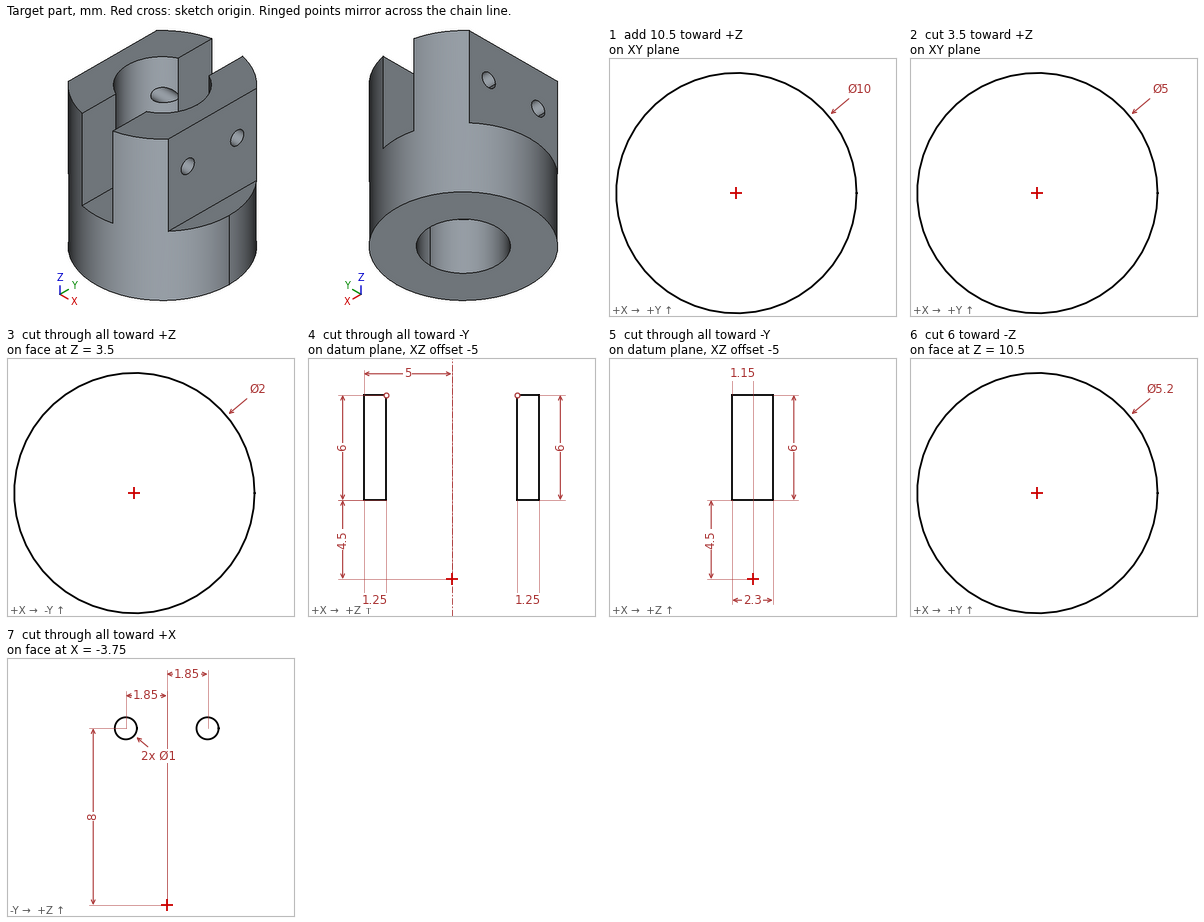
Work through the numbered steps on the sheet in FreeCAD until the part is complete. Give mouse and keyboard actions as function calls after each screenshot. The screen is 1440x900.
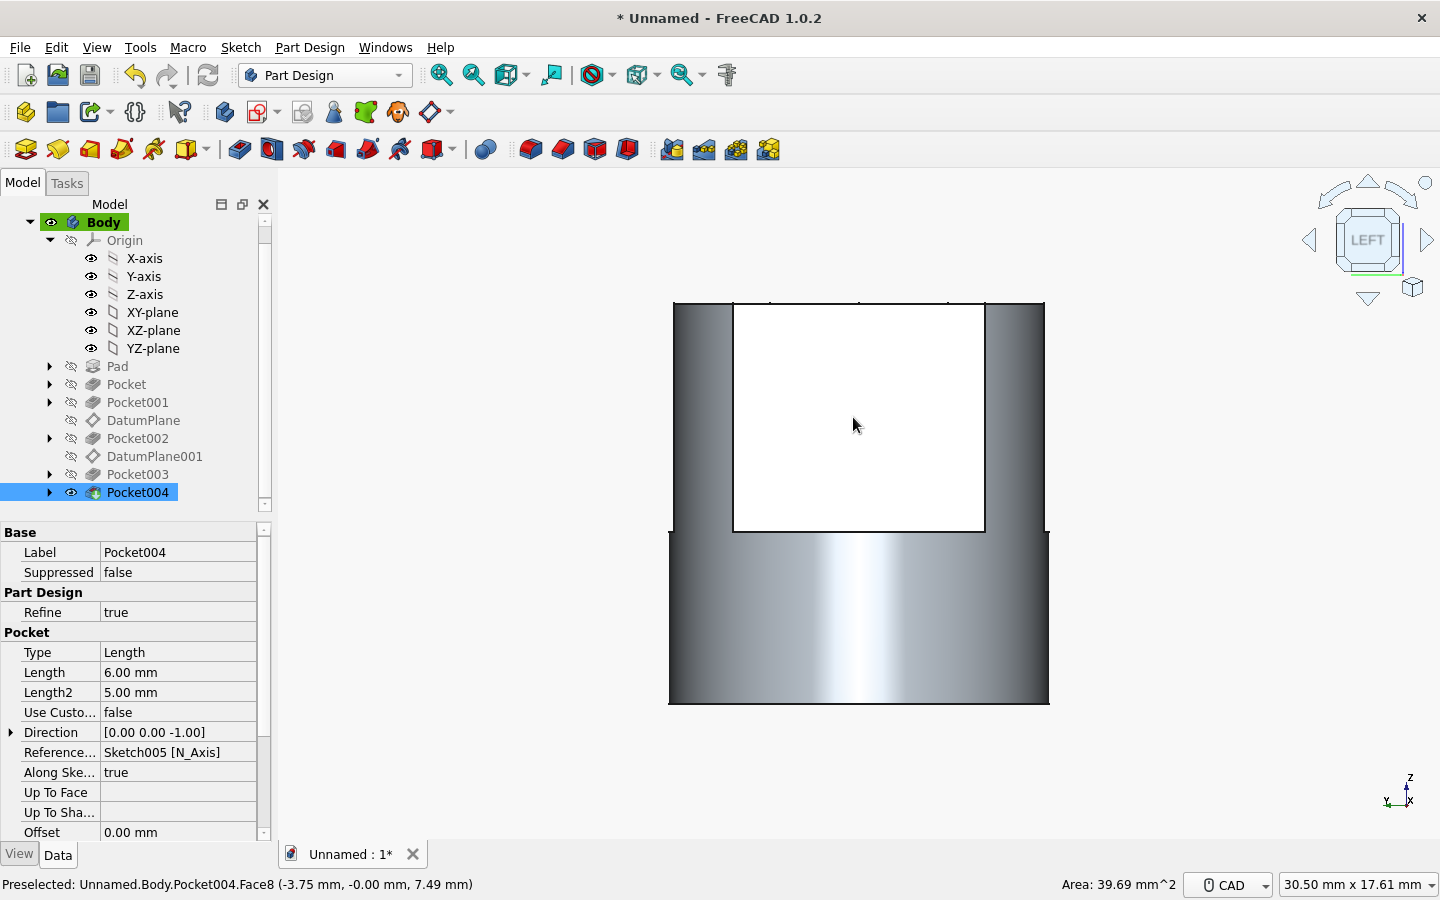
click(258, 112)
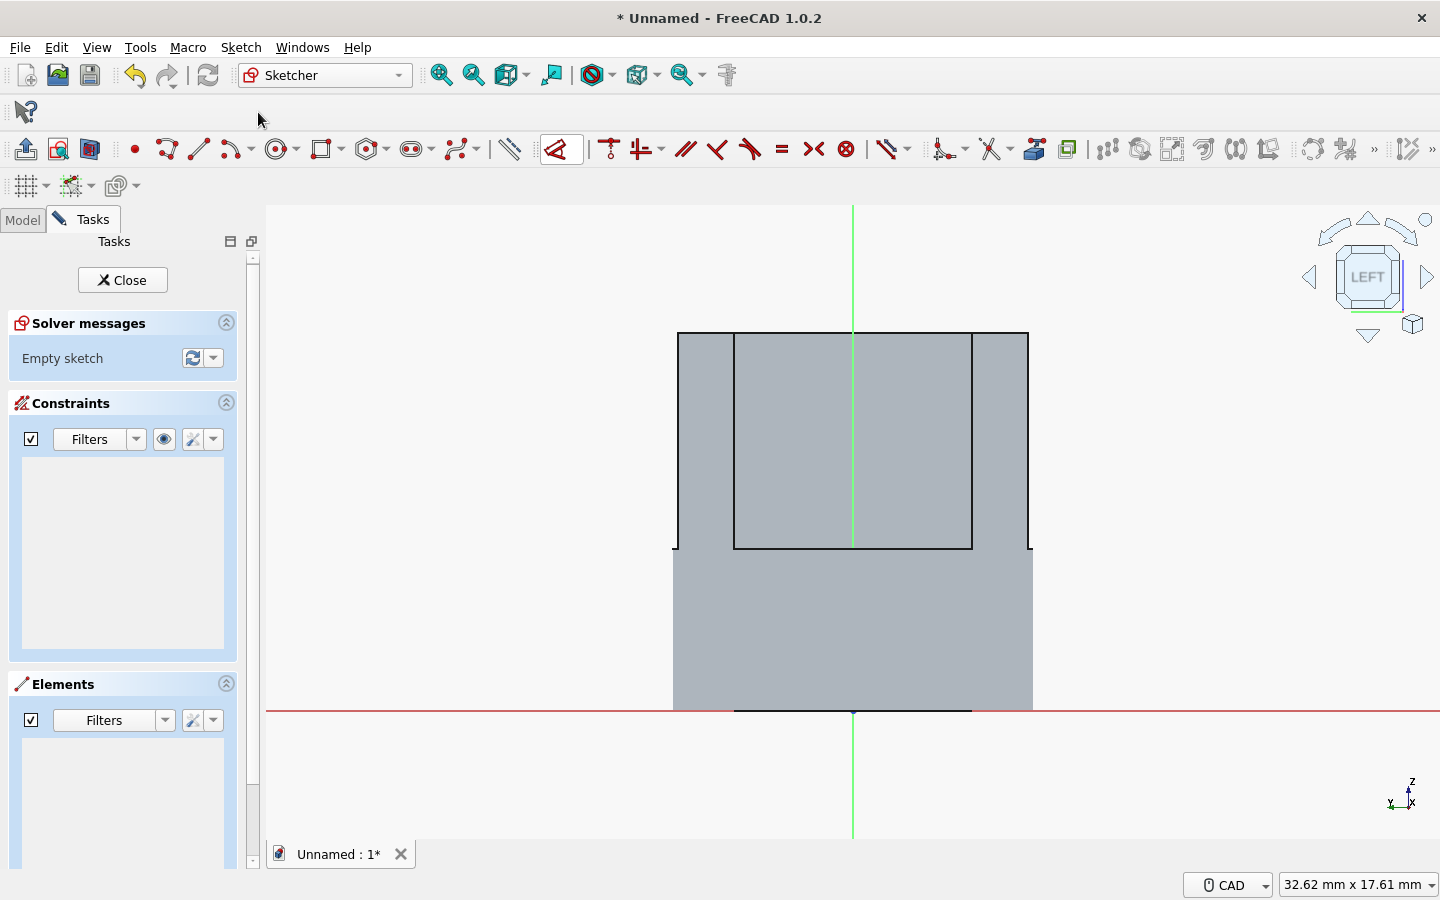
key(g)
key(c)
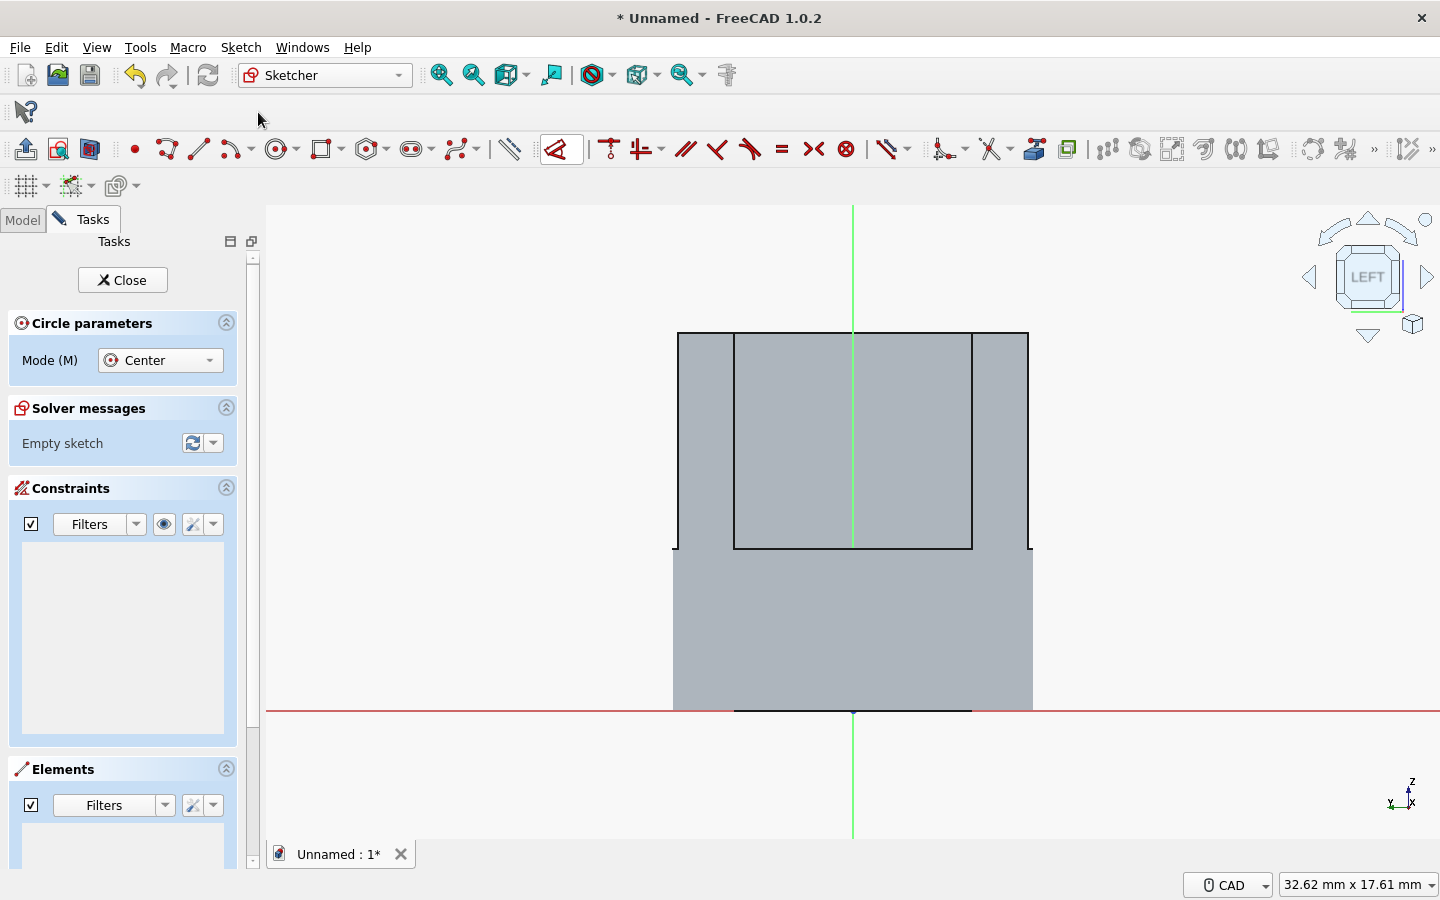
scroll(786, 423, up, 2)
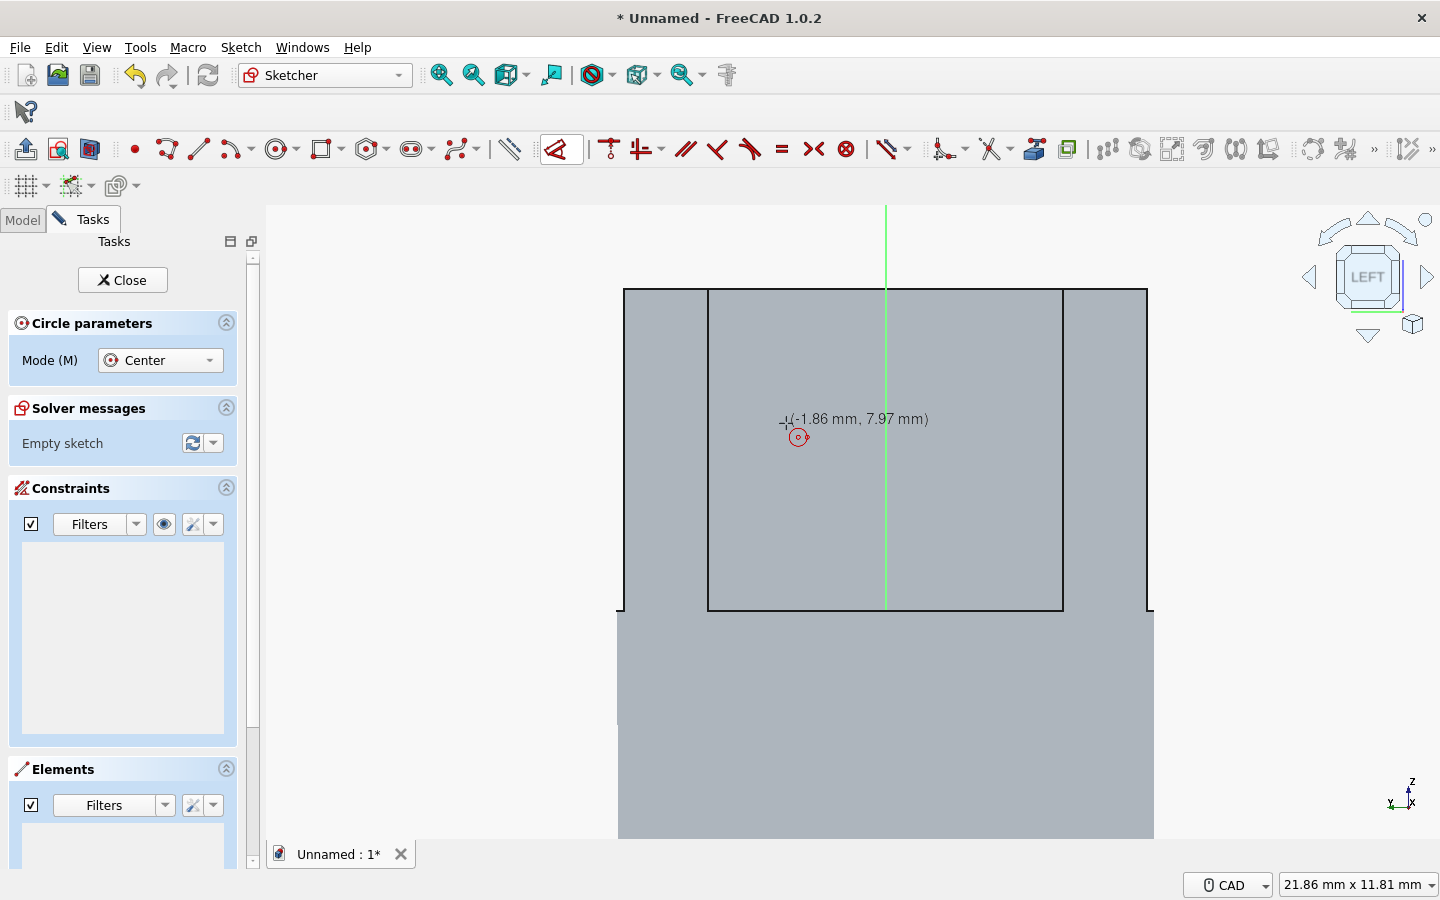
click(786, 423)
move(805, 404)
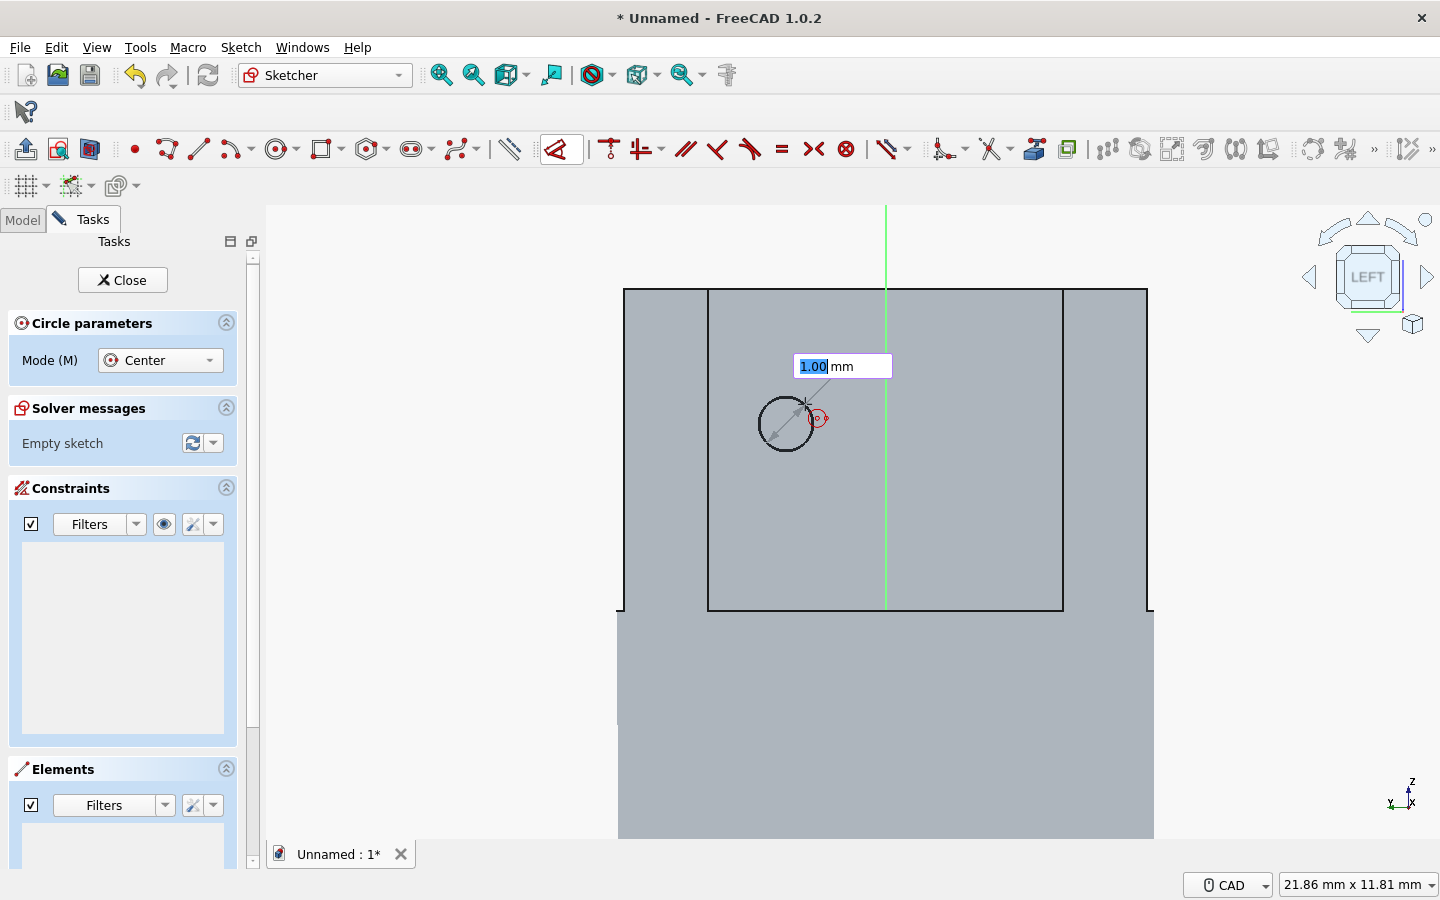
text(1)
key(Return)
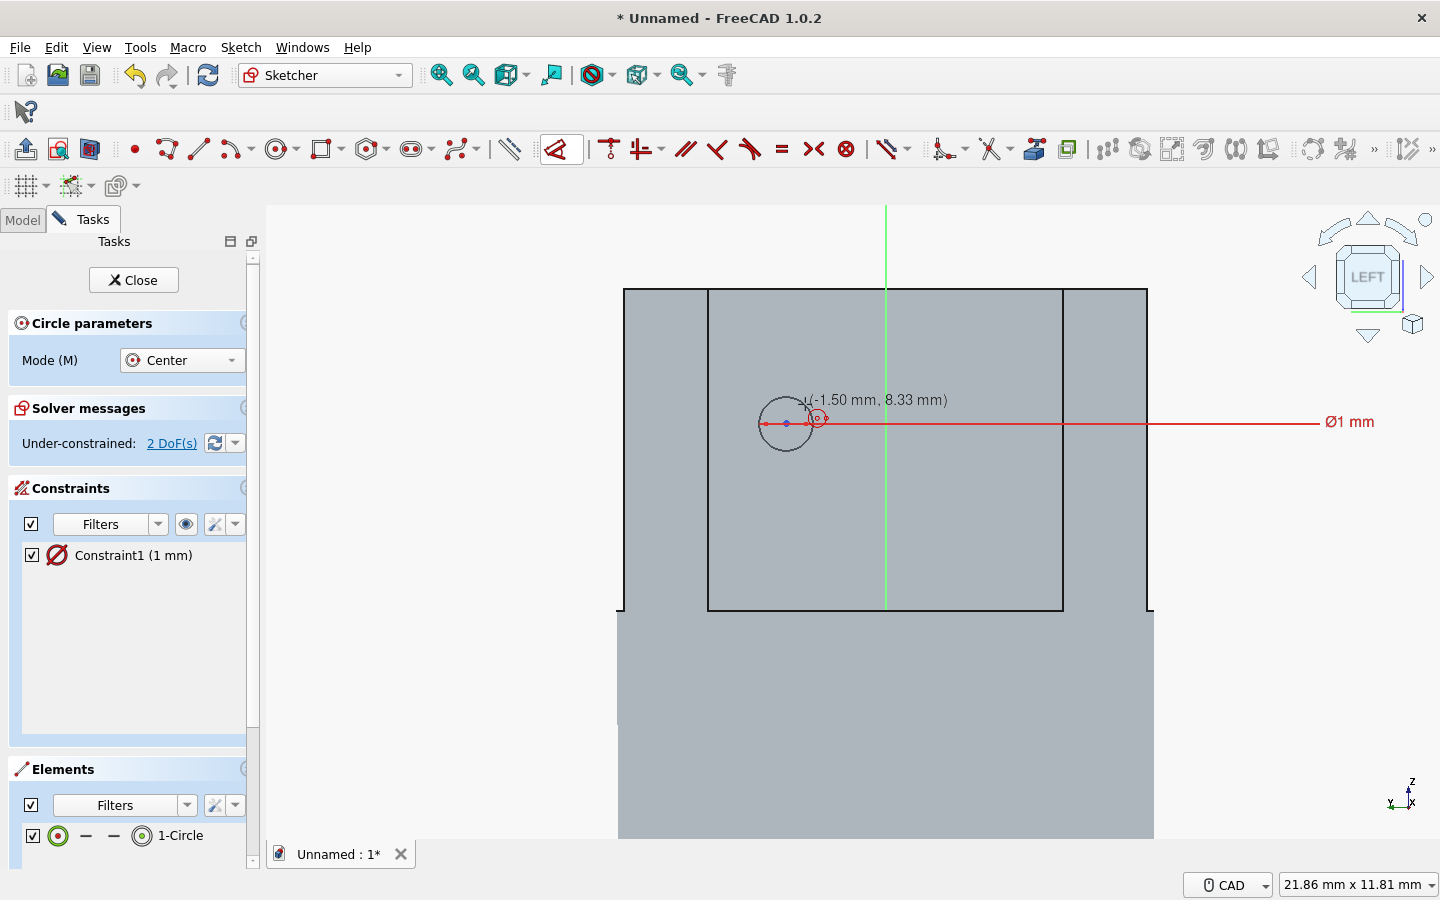
click(985, 423)
move(1004, 404)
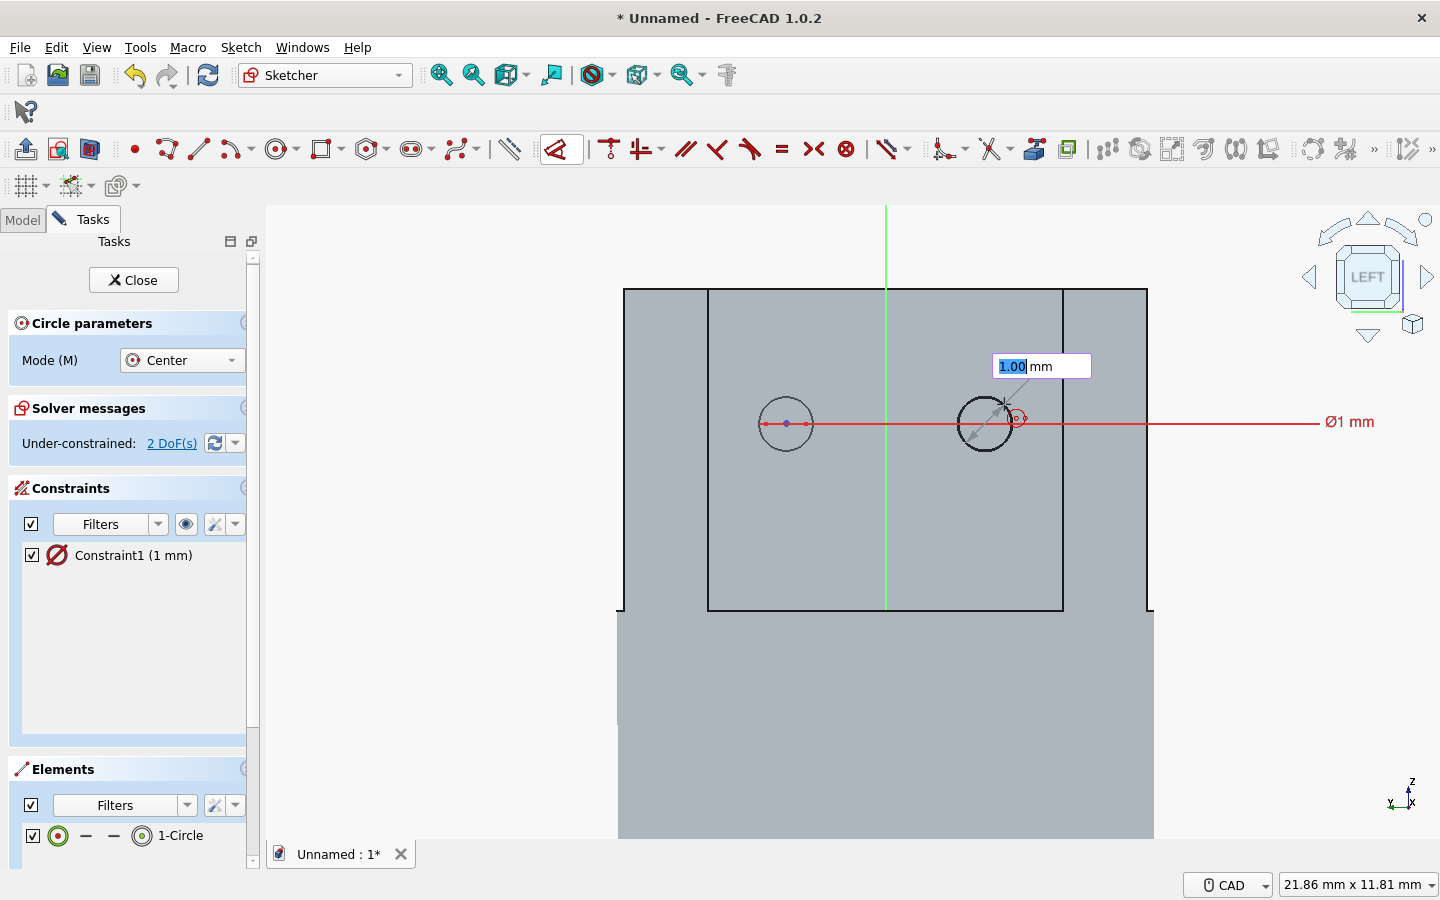
text(1)
key(Return)
key(Escape)